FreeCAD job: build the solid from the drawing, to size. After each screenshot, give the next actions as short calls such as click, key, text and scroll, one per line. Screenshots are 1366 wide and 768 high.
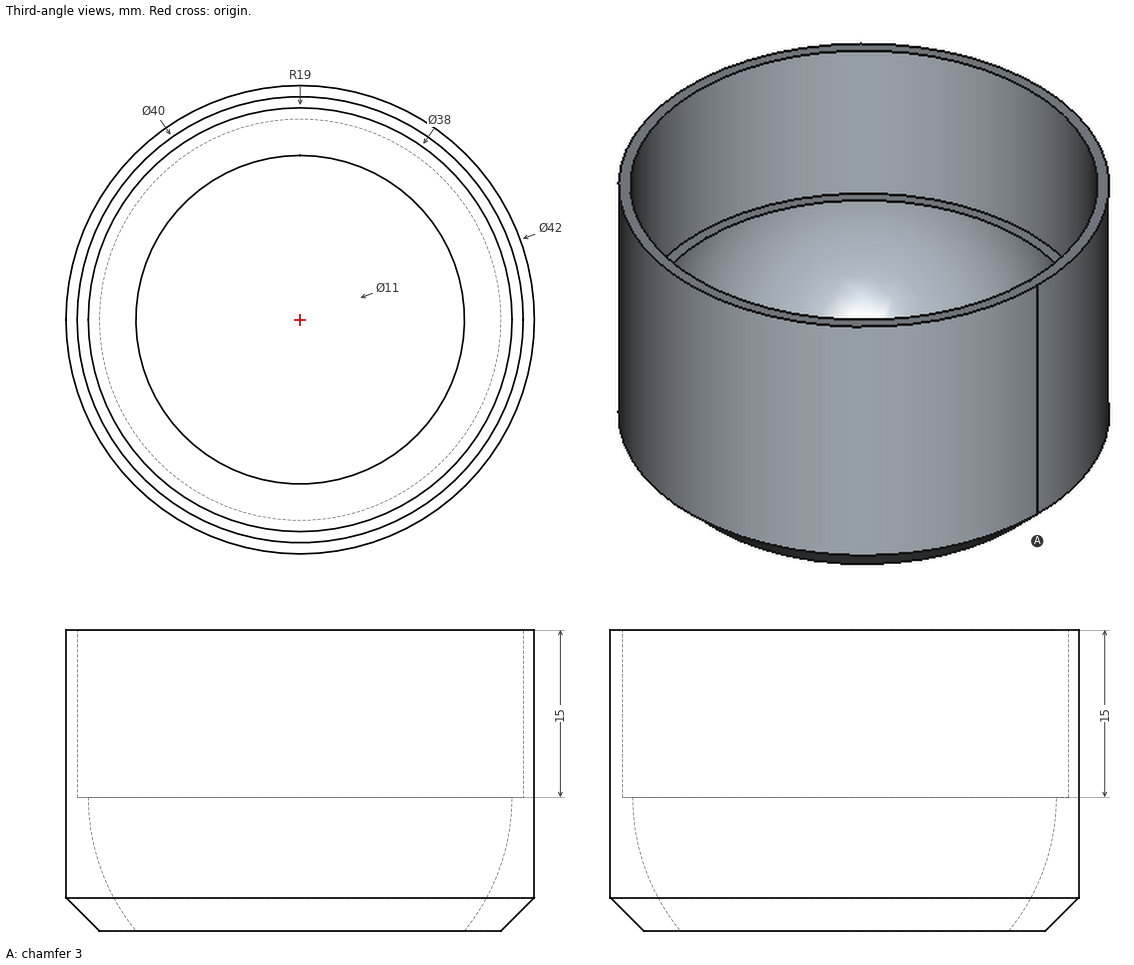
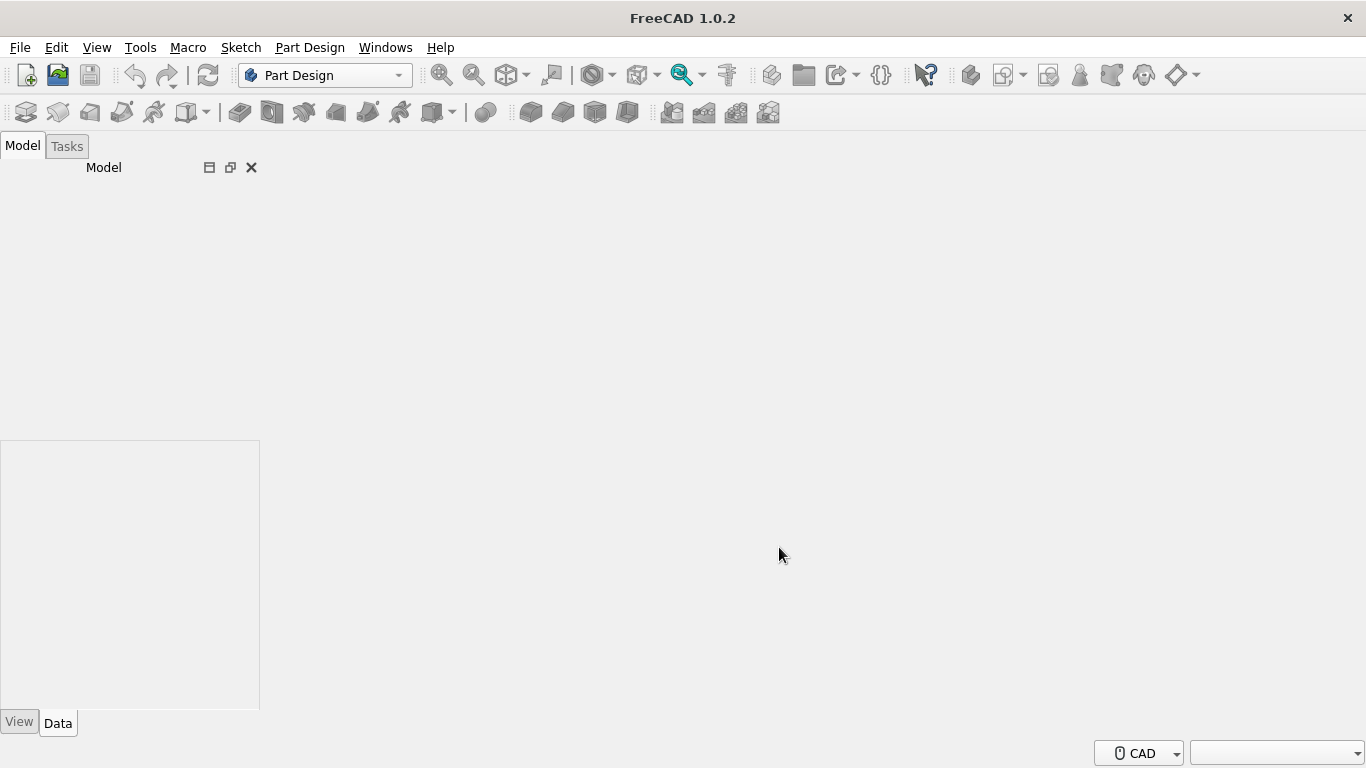
click(26, 76)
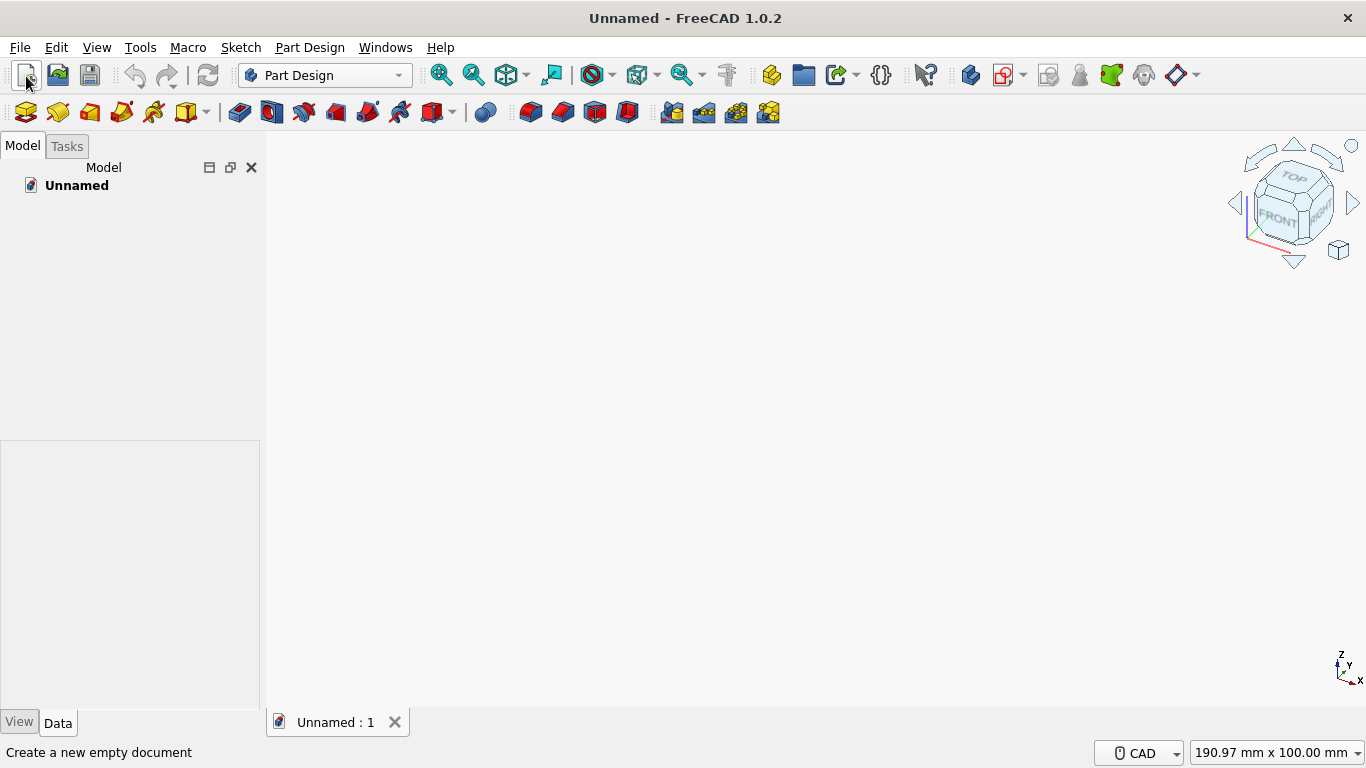
click(1004, 76)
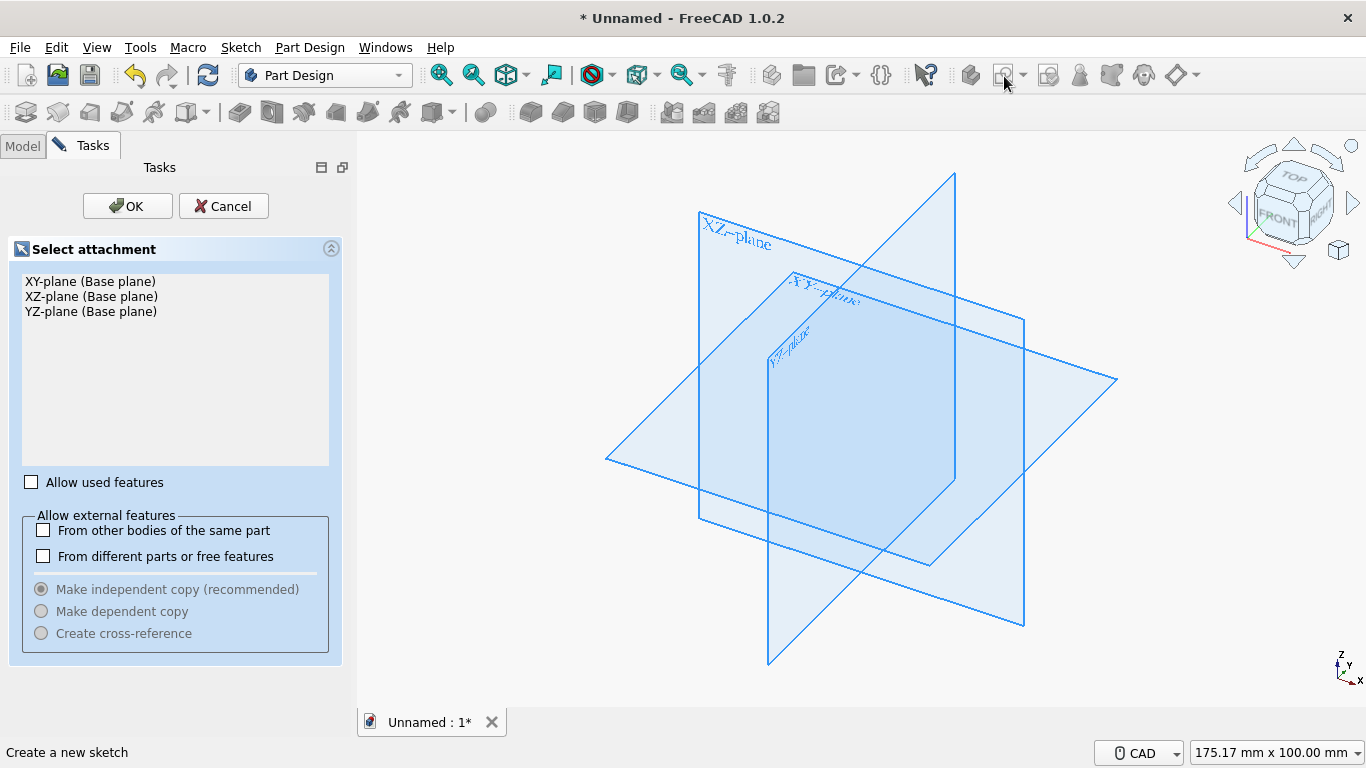
click(82, 282)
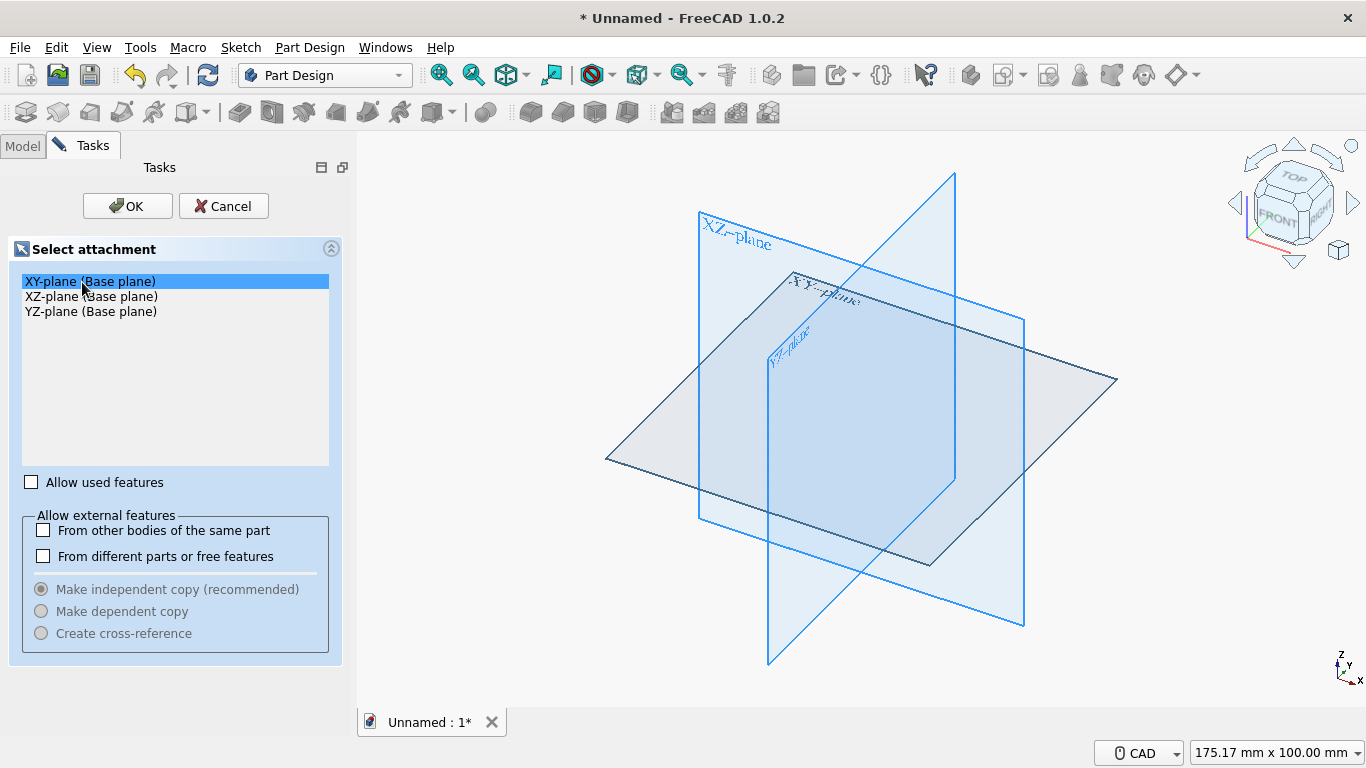
click(128, 206)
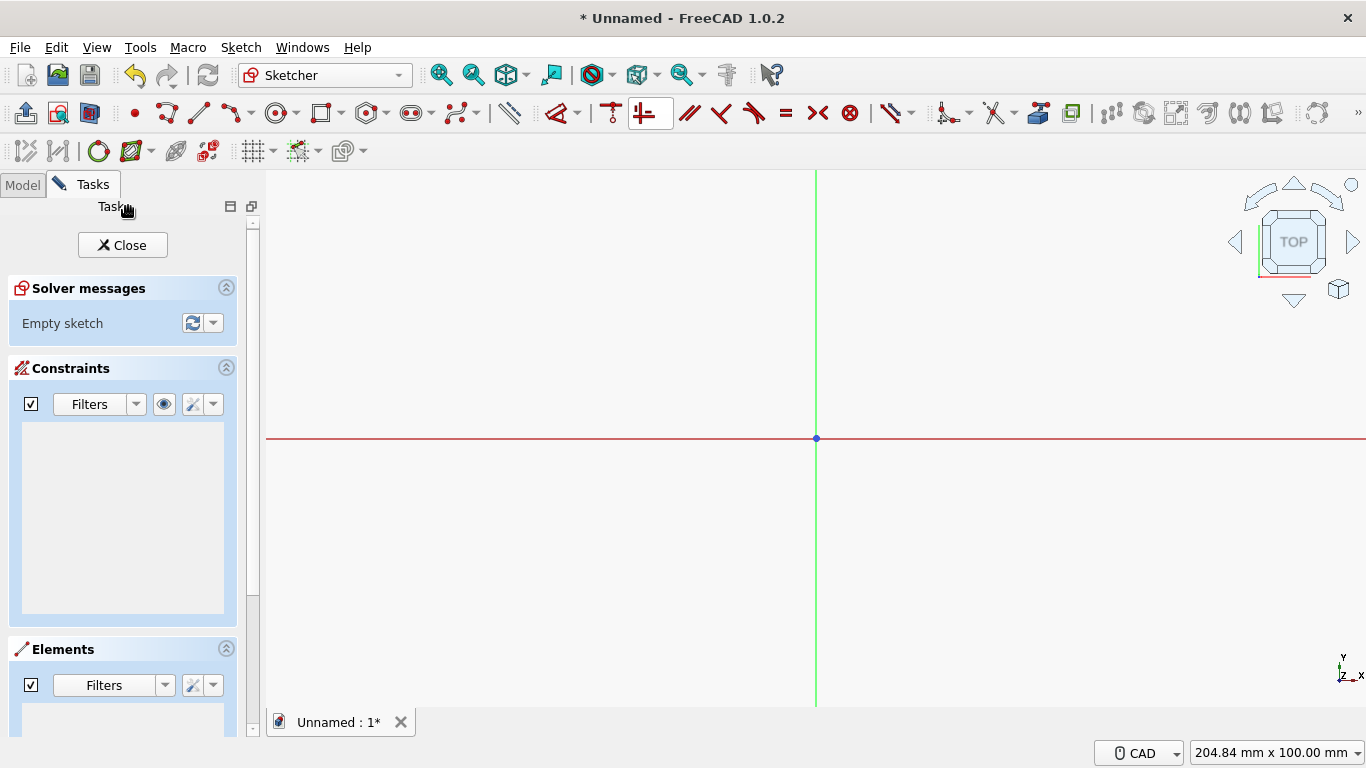
scroll(955, 439, up, 2)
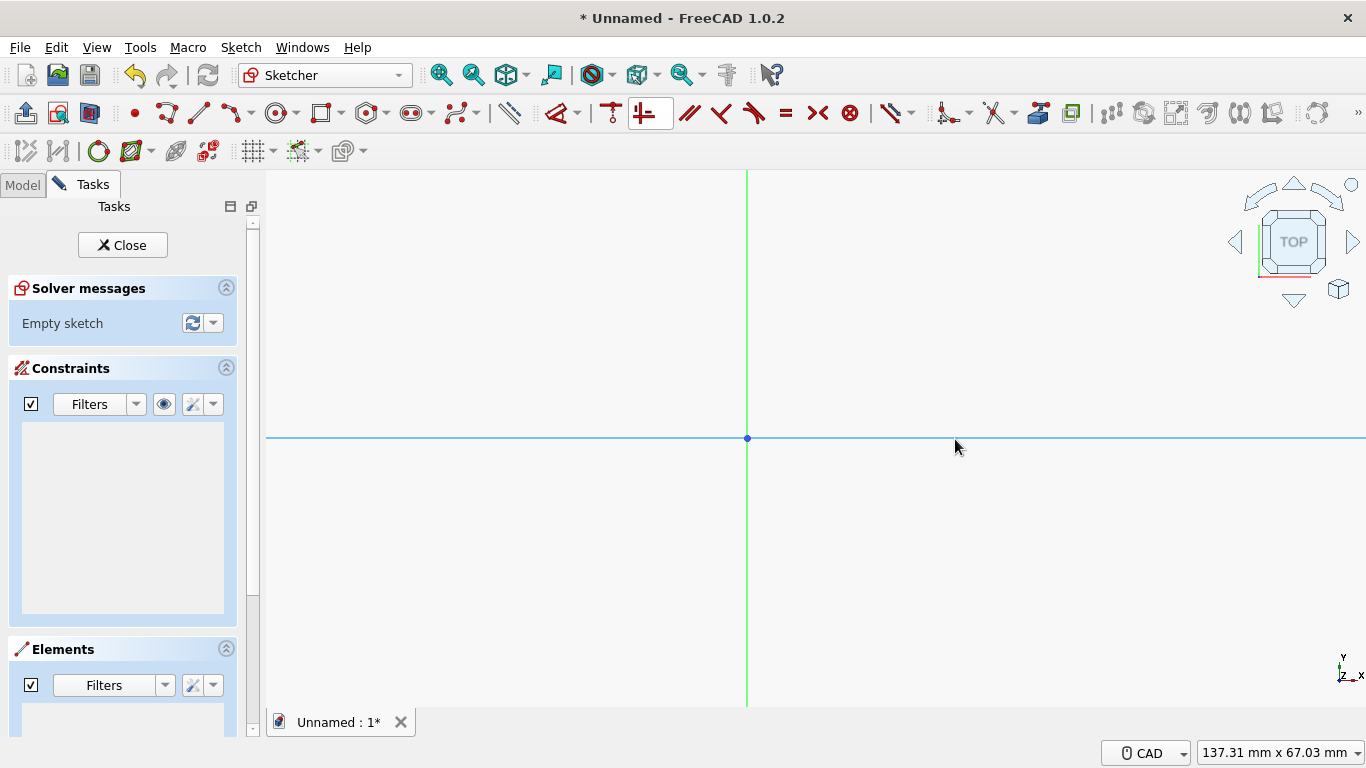
click(276, 114)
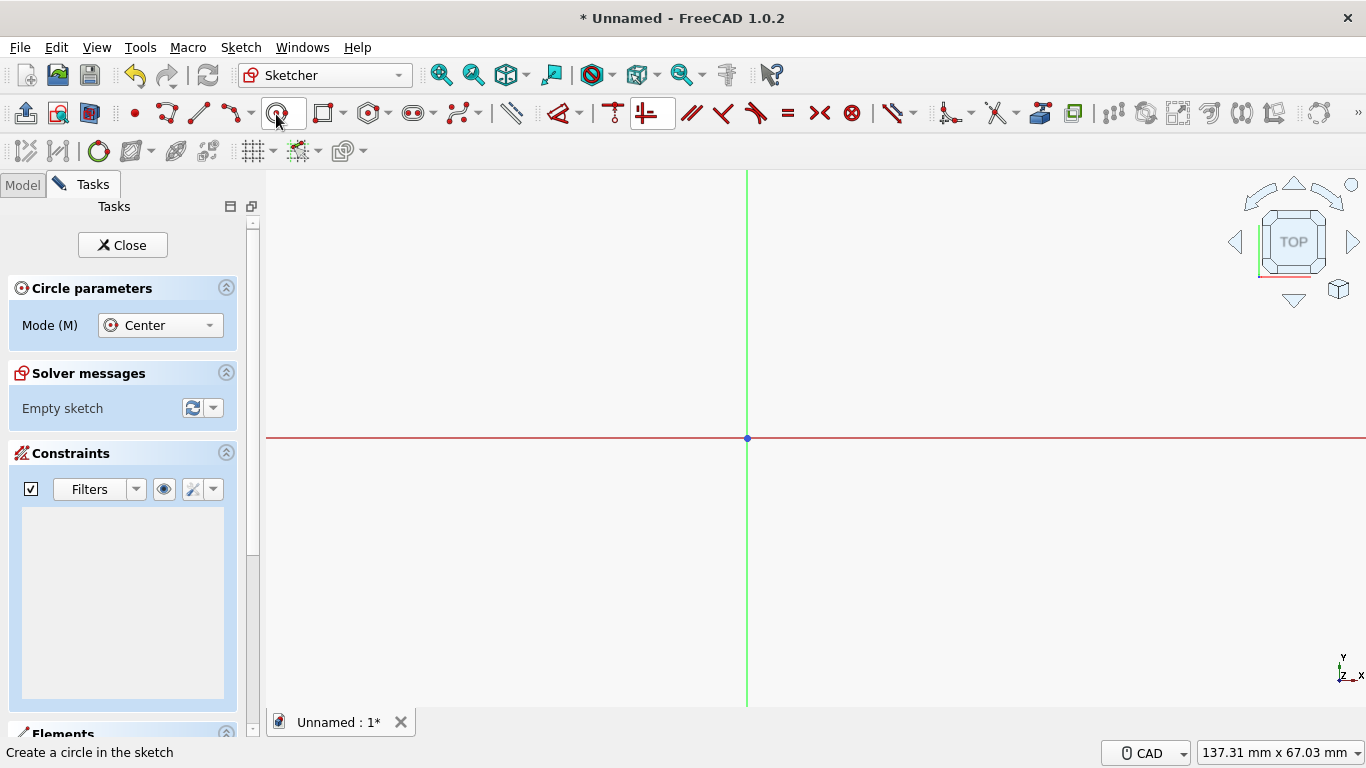
click(747, 438)
move(866, 319)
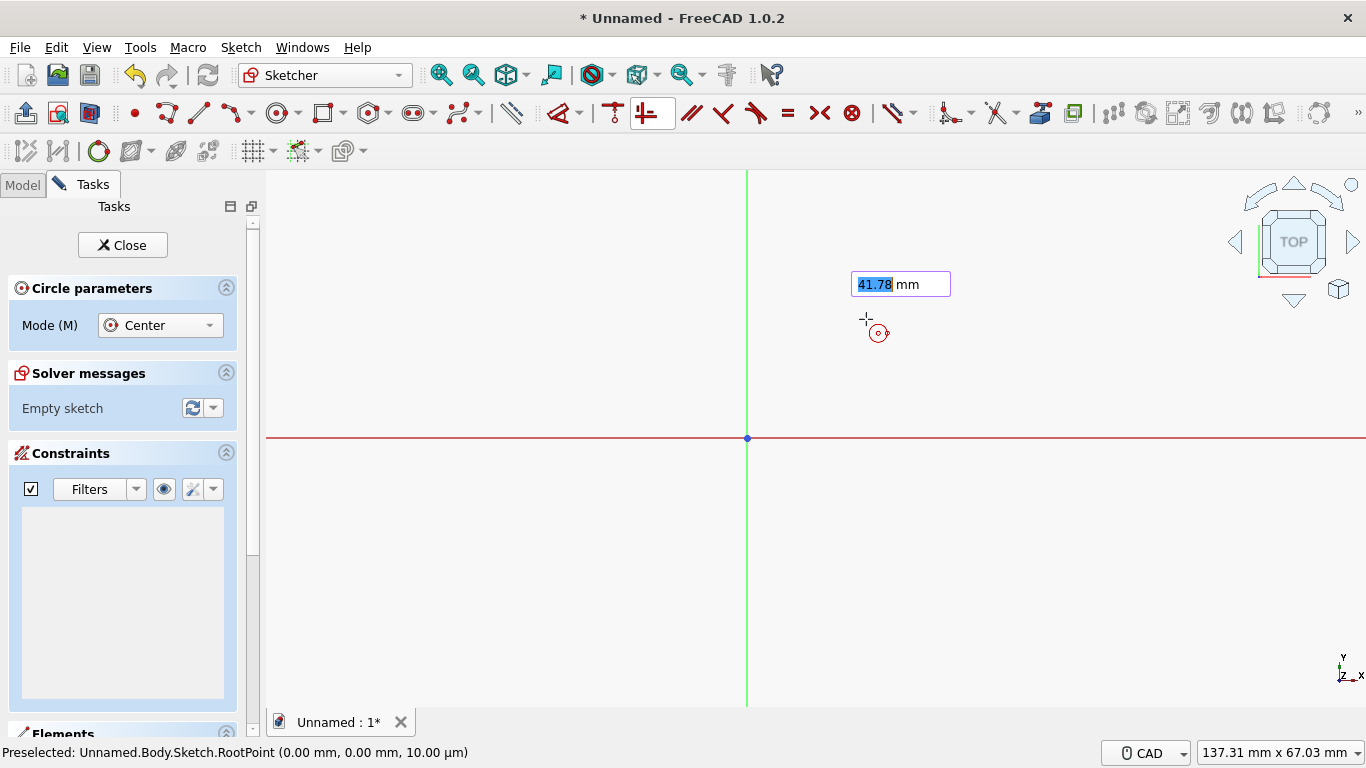
text(42)
key(Return)
key(Escape)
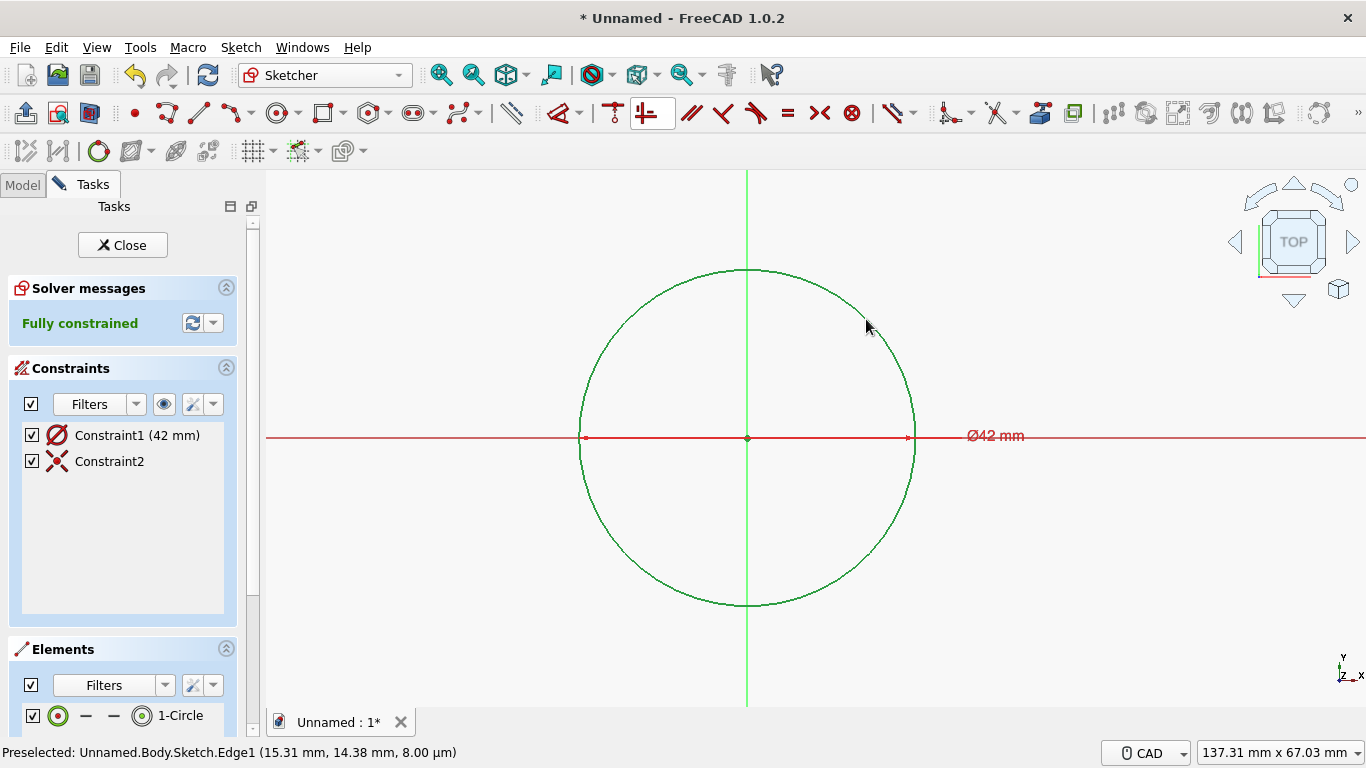
click(123, 245)